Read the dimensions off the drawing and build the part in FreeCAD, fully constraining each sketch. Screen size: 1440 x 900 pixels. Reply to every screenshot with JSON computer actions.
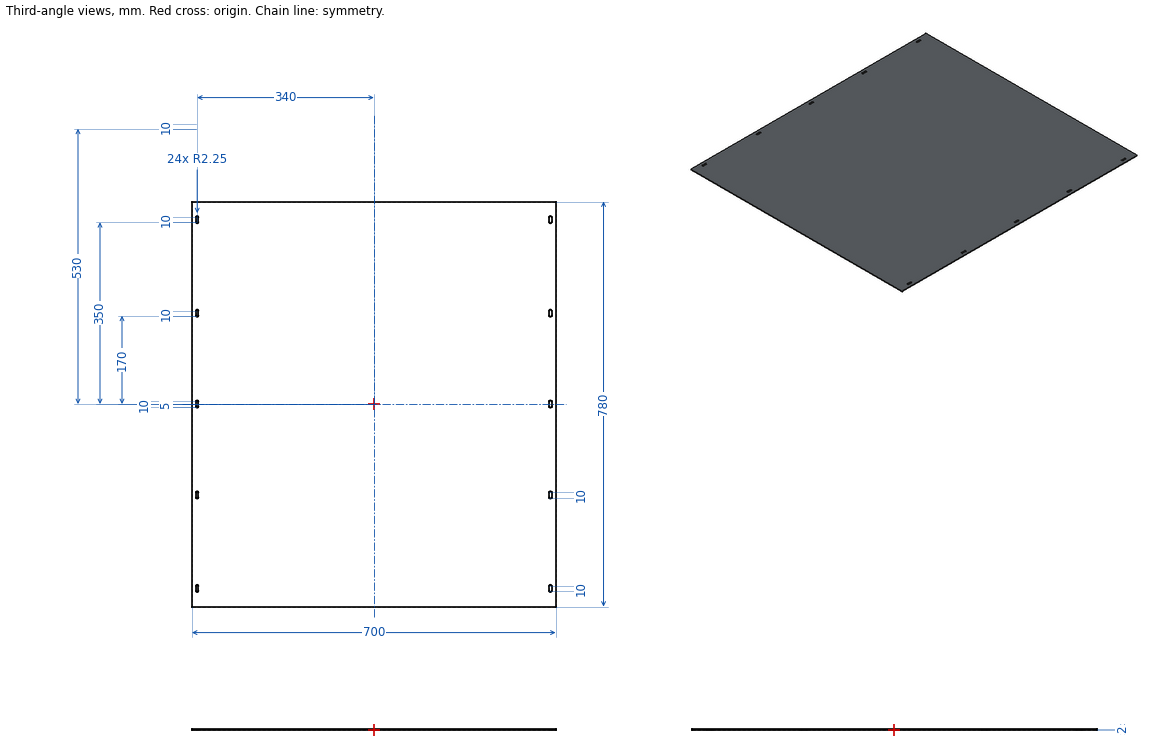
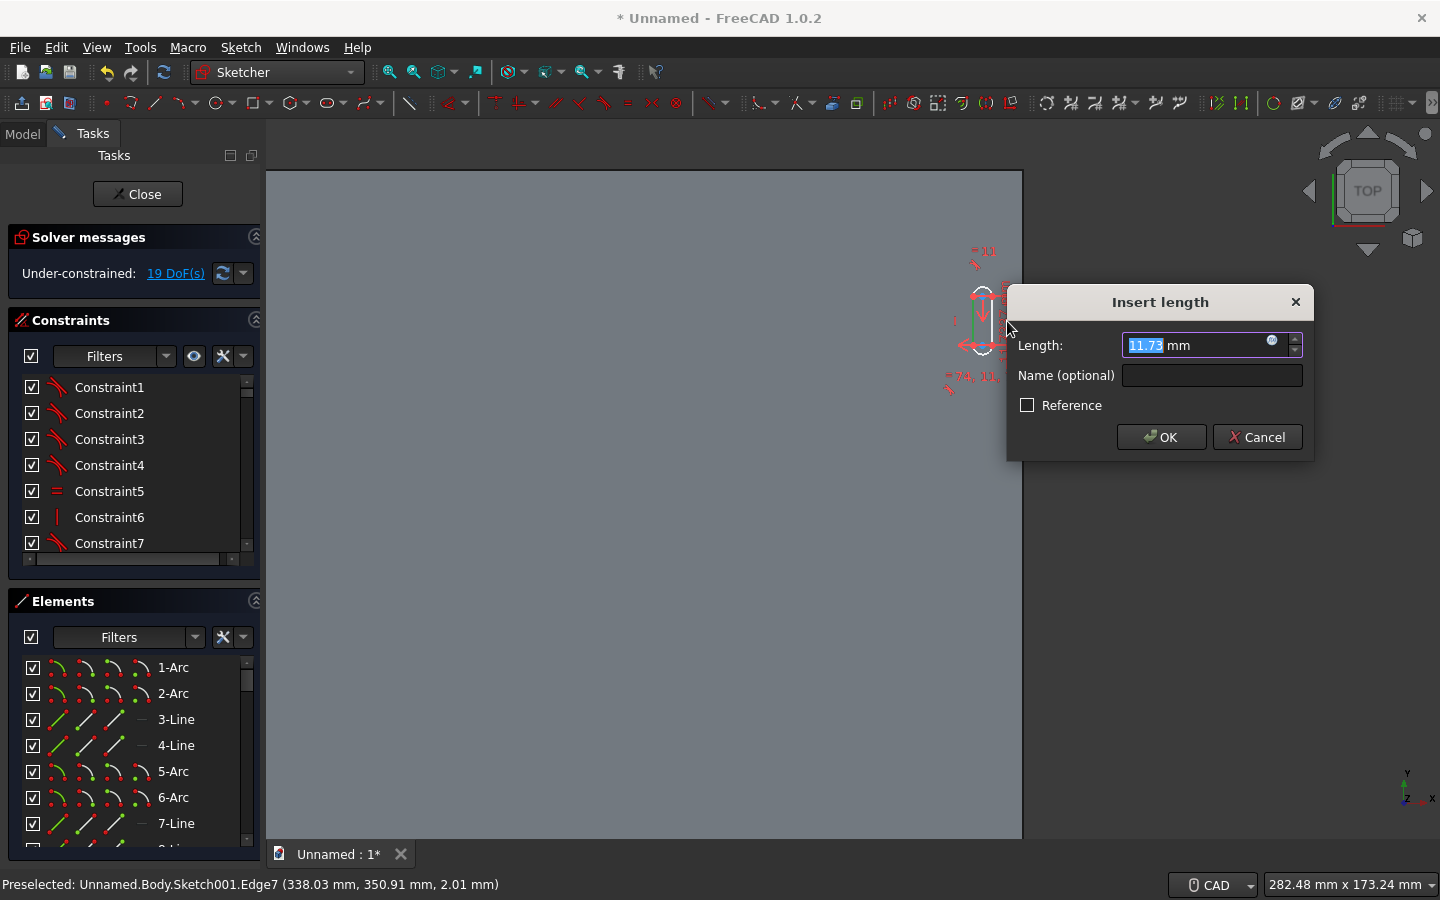
{"action": "type", "text": "10"}
{"action": "key", "text": "Return"}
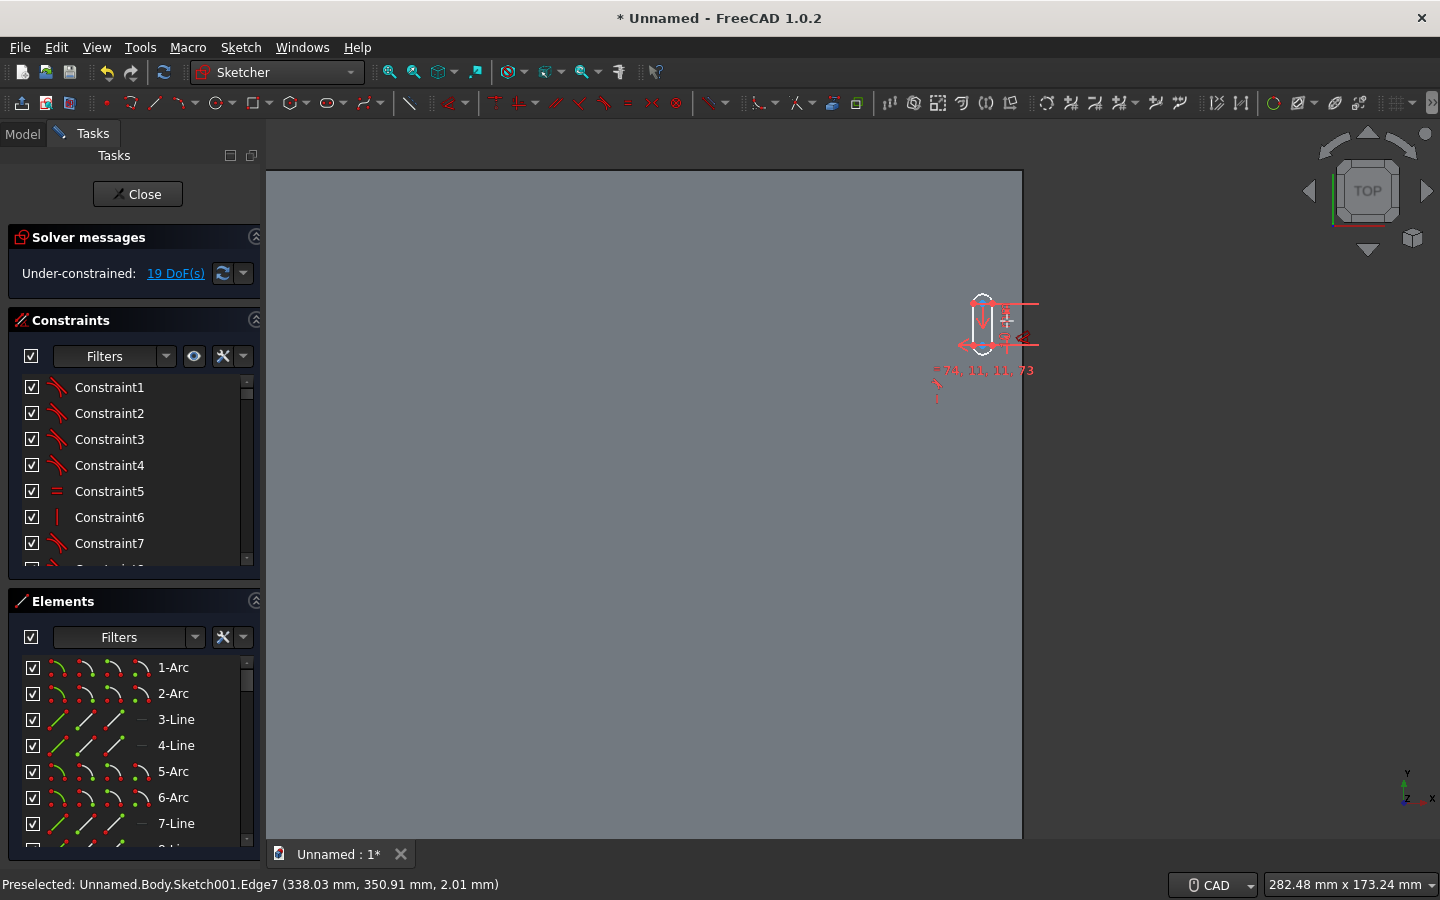
{"action": "scroll", "coordinate": [975, 332], "scroll_direction": "down", "scroll_amount": 10}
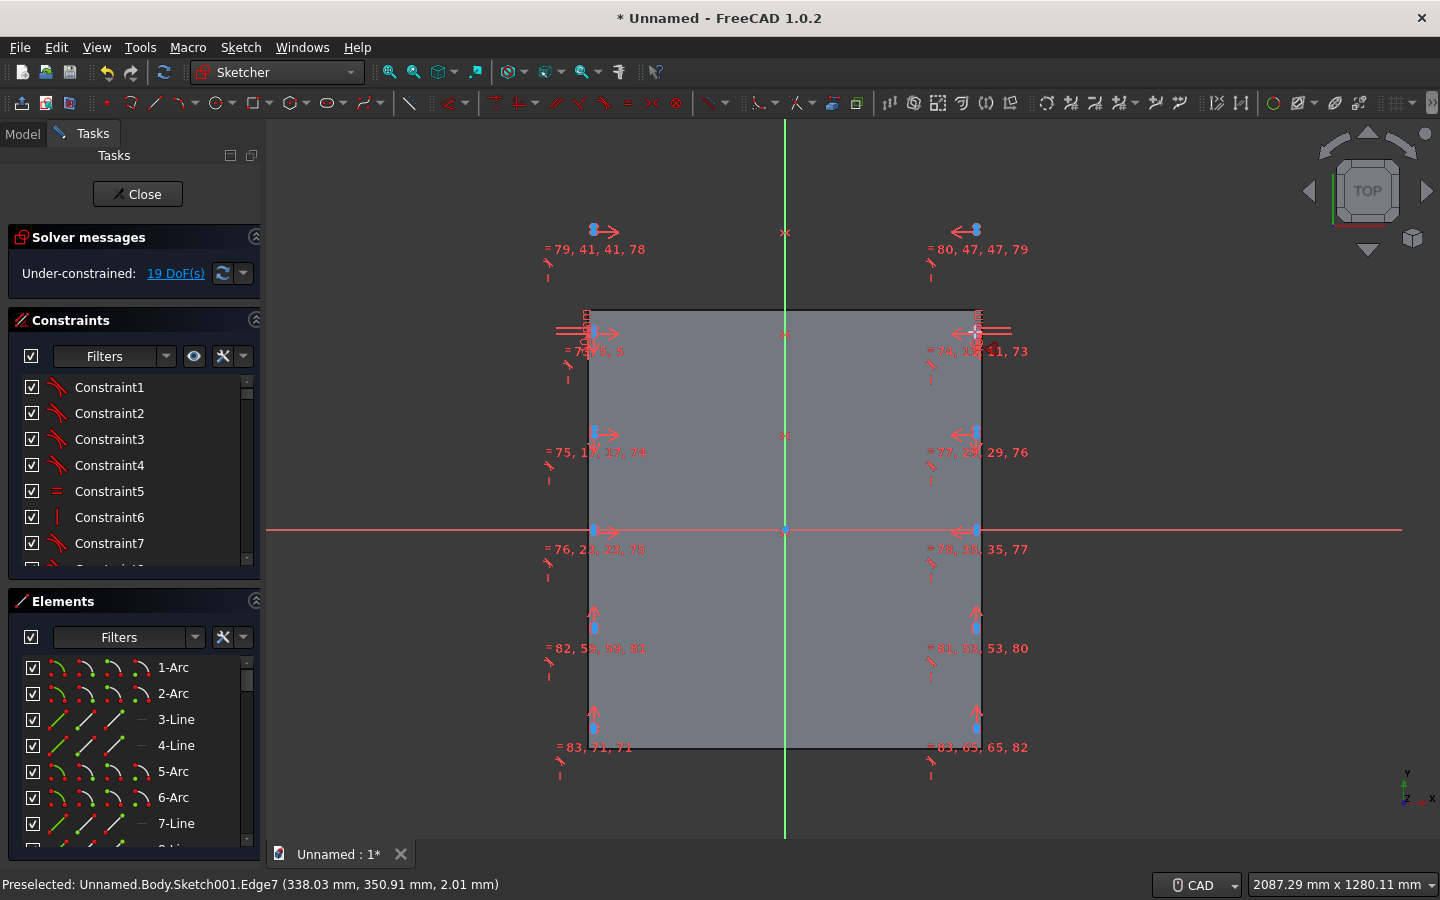
{"action": "scroll", "coordinate": [593, 433], "scroll_direction": "up", "scroll_amount": 10}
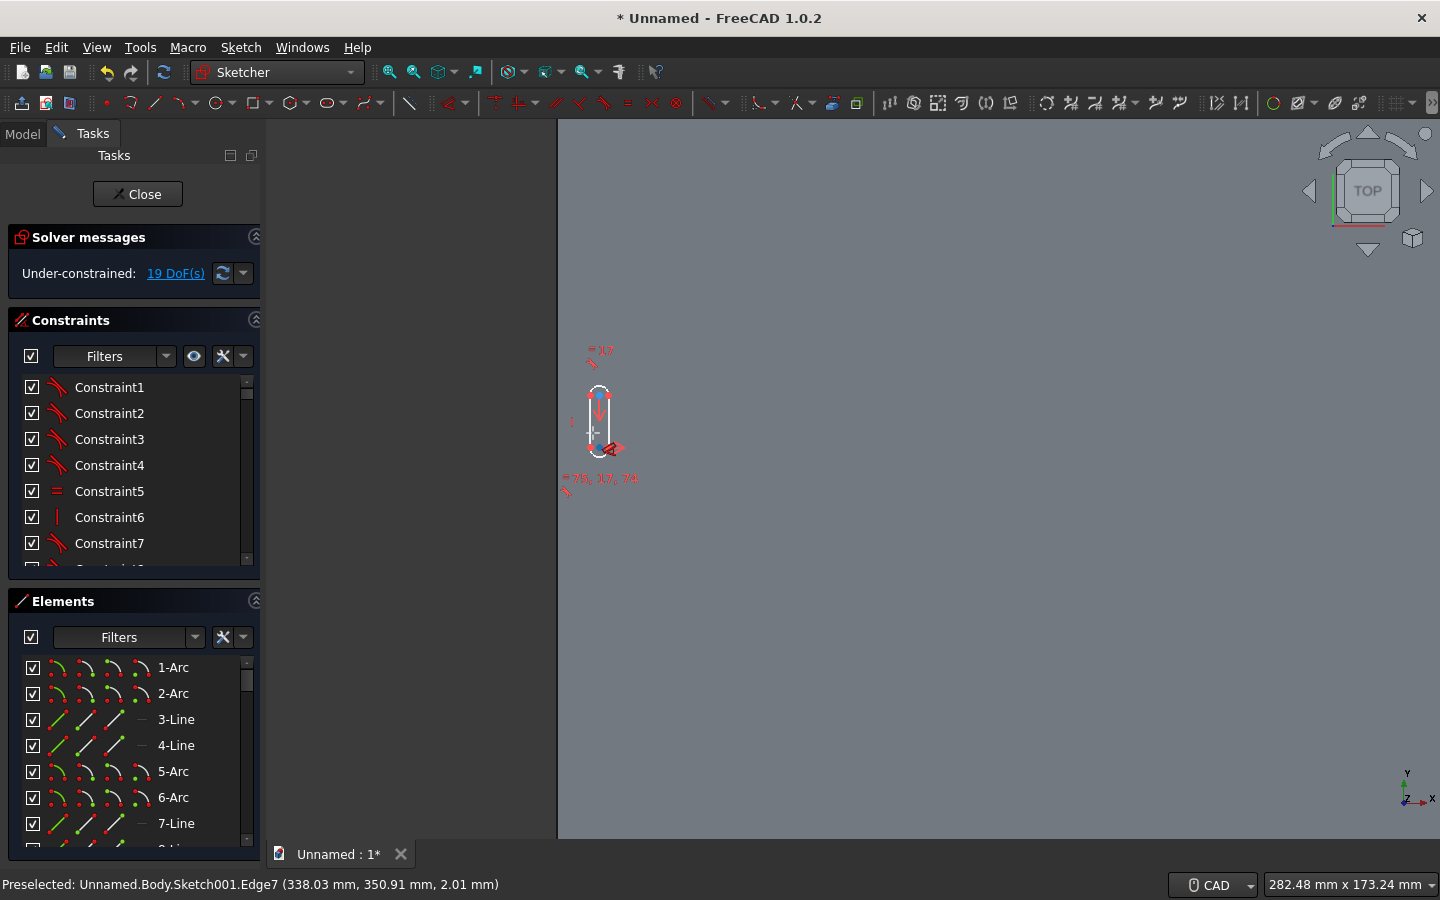
{"action": "left_click", "coordinate": [590, 432]}
{"action": "left_click", "coordinate": [556, 422]}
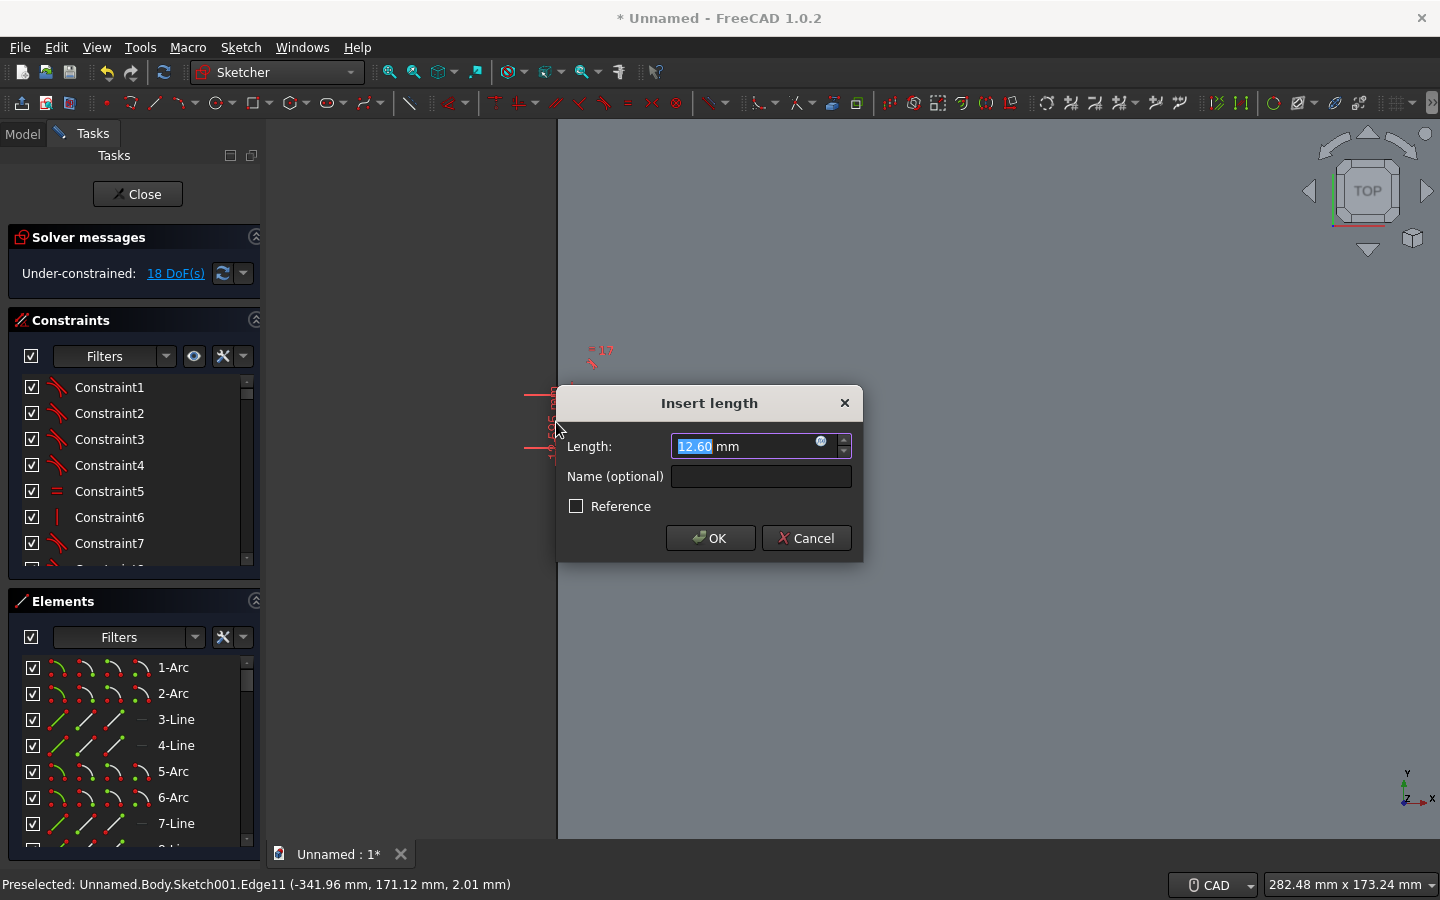
{"action": "type", "text": "10"}
{"action": "key", "text": "Return"}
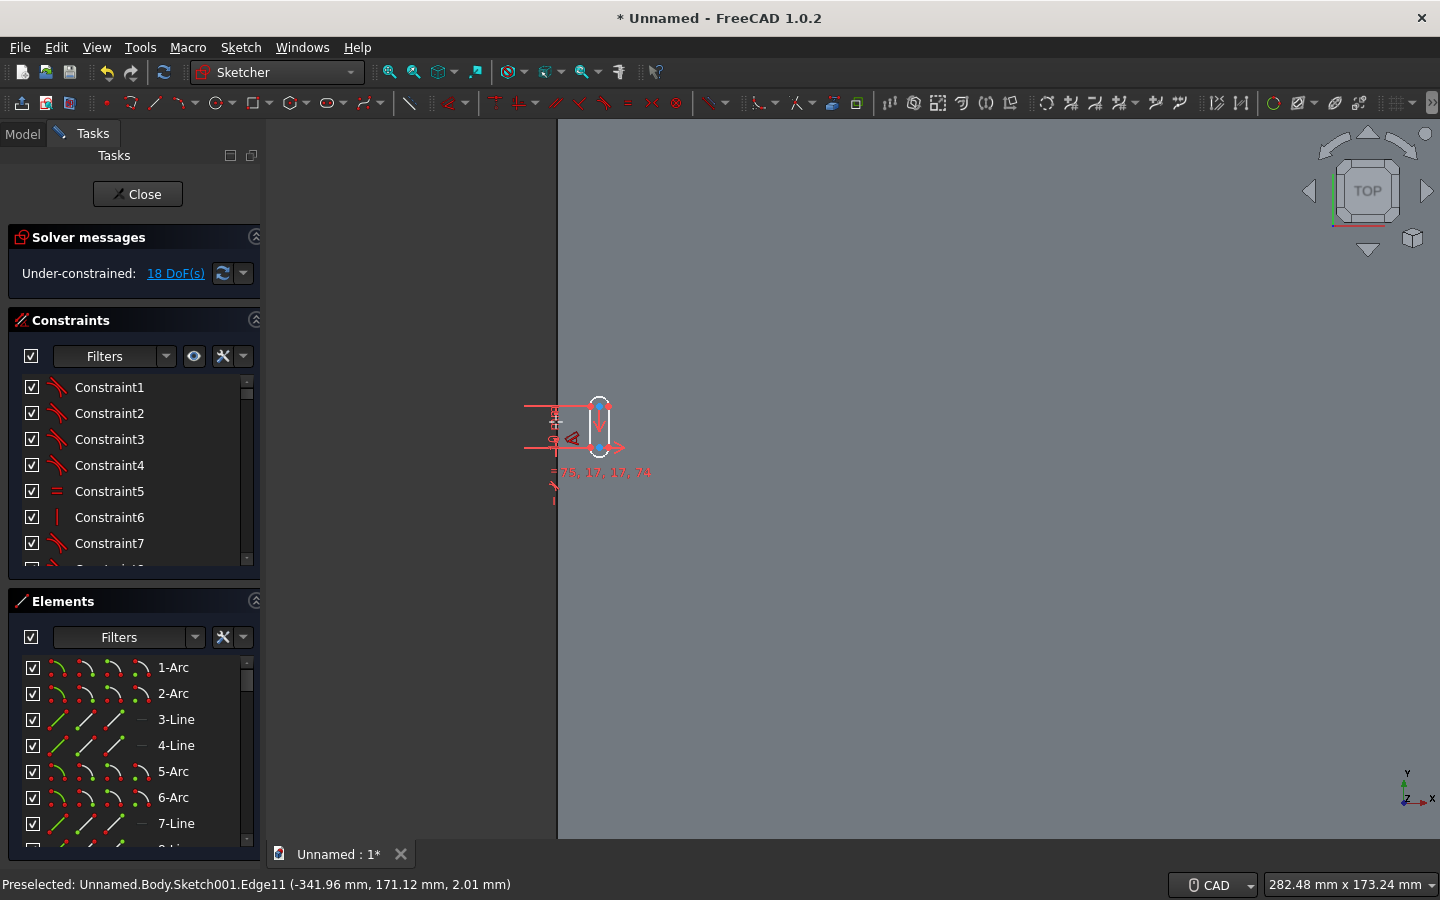
{"action": "scroll", "coordinate": [592, 433], "scroll_direction": "down", "scroll_amount": 10}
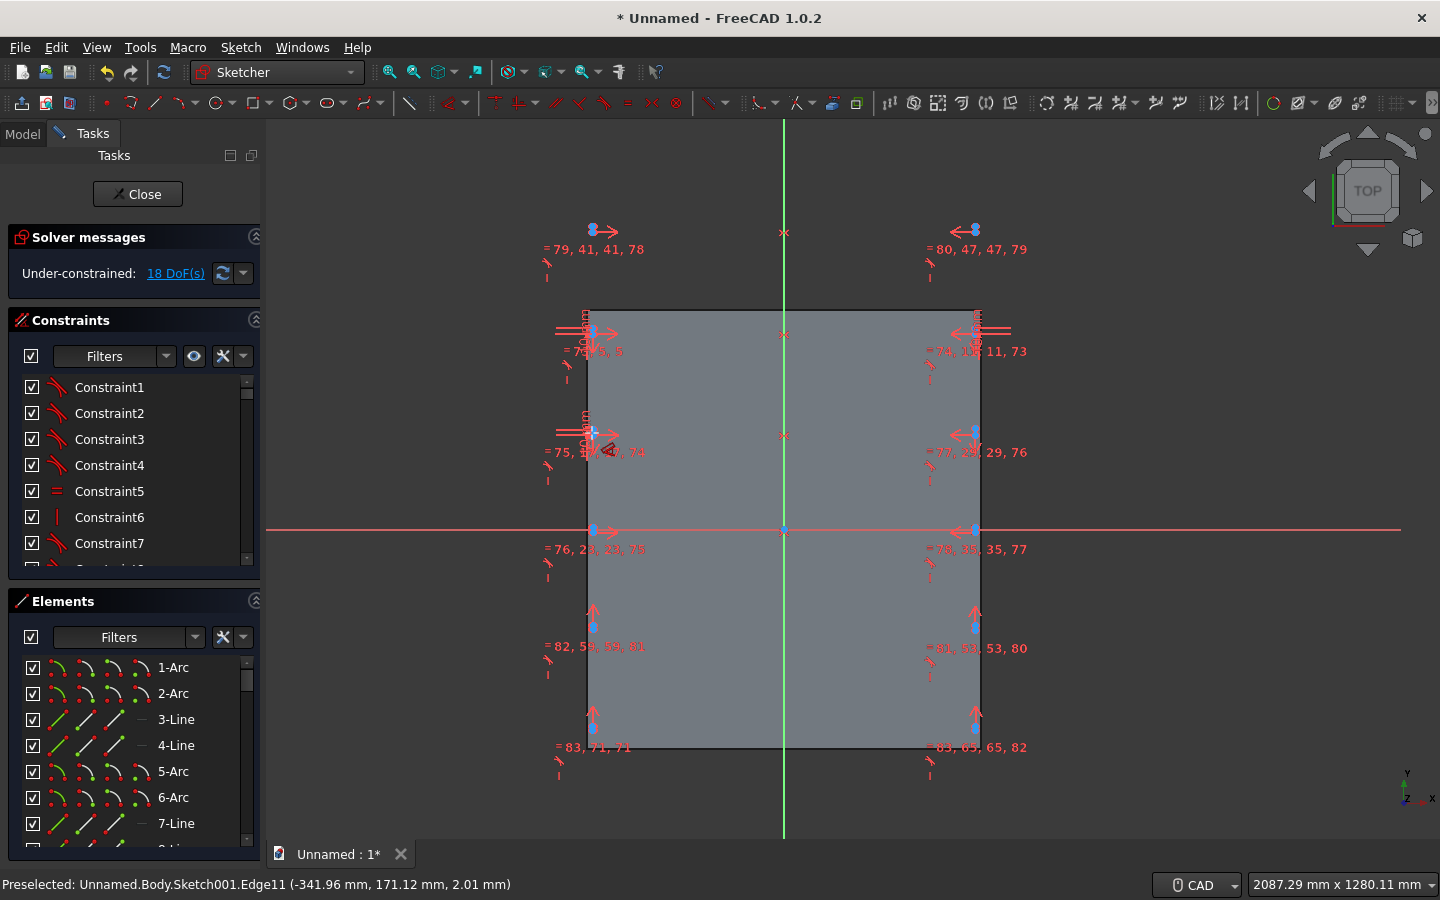
{"action": "scroll", "coordinate": [592, 531], "scroll_direction": "up", "scroll_amount": 12}